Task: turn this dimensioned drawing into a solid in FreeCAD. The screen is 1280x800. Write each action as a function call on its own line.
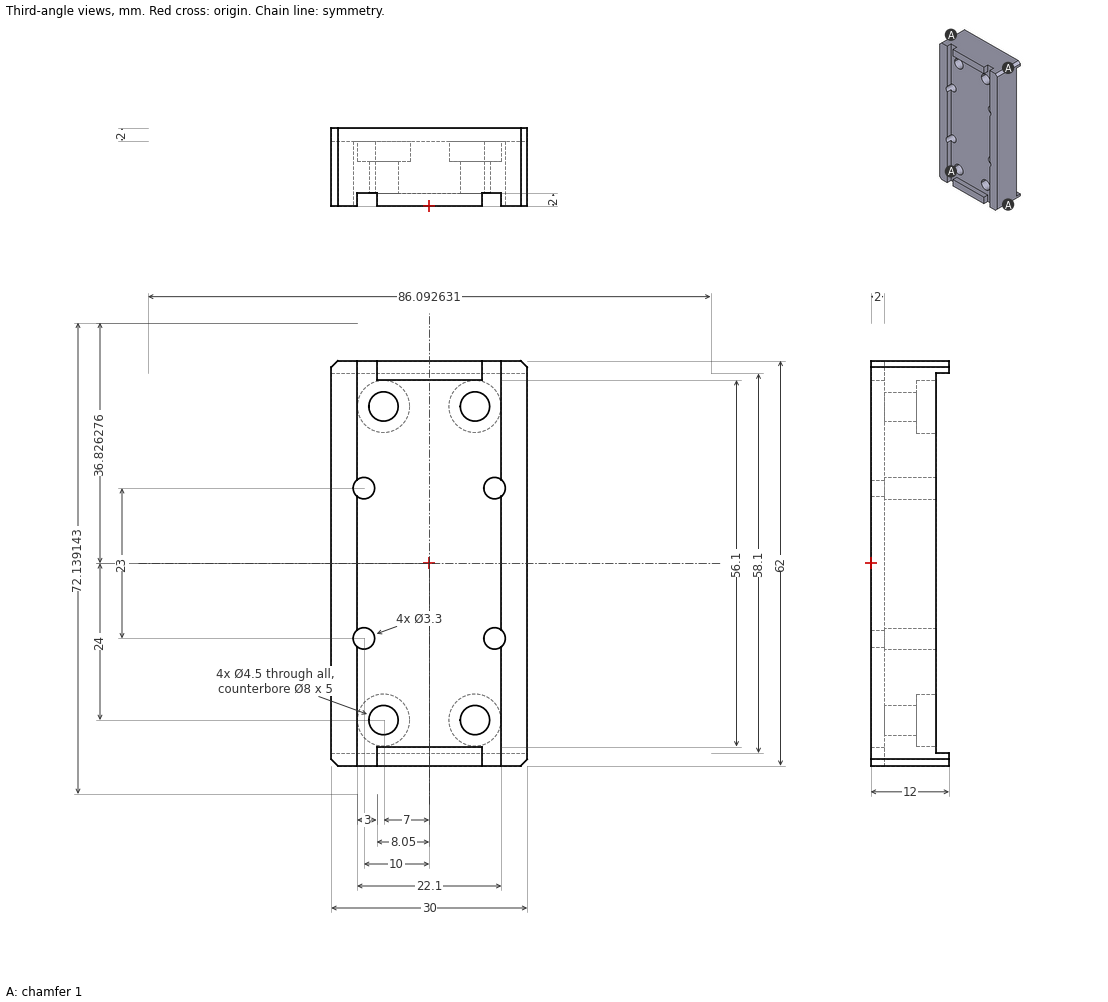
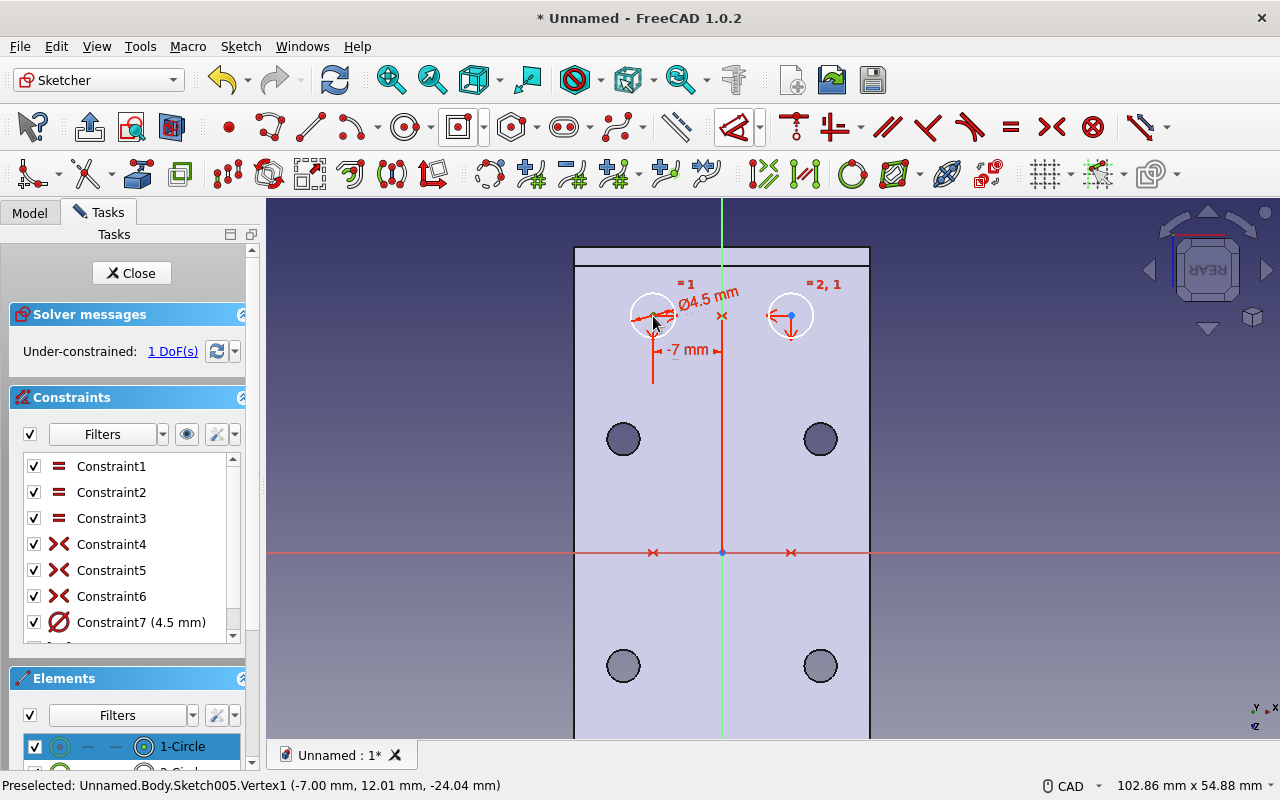
click(760, 128)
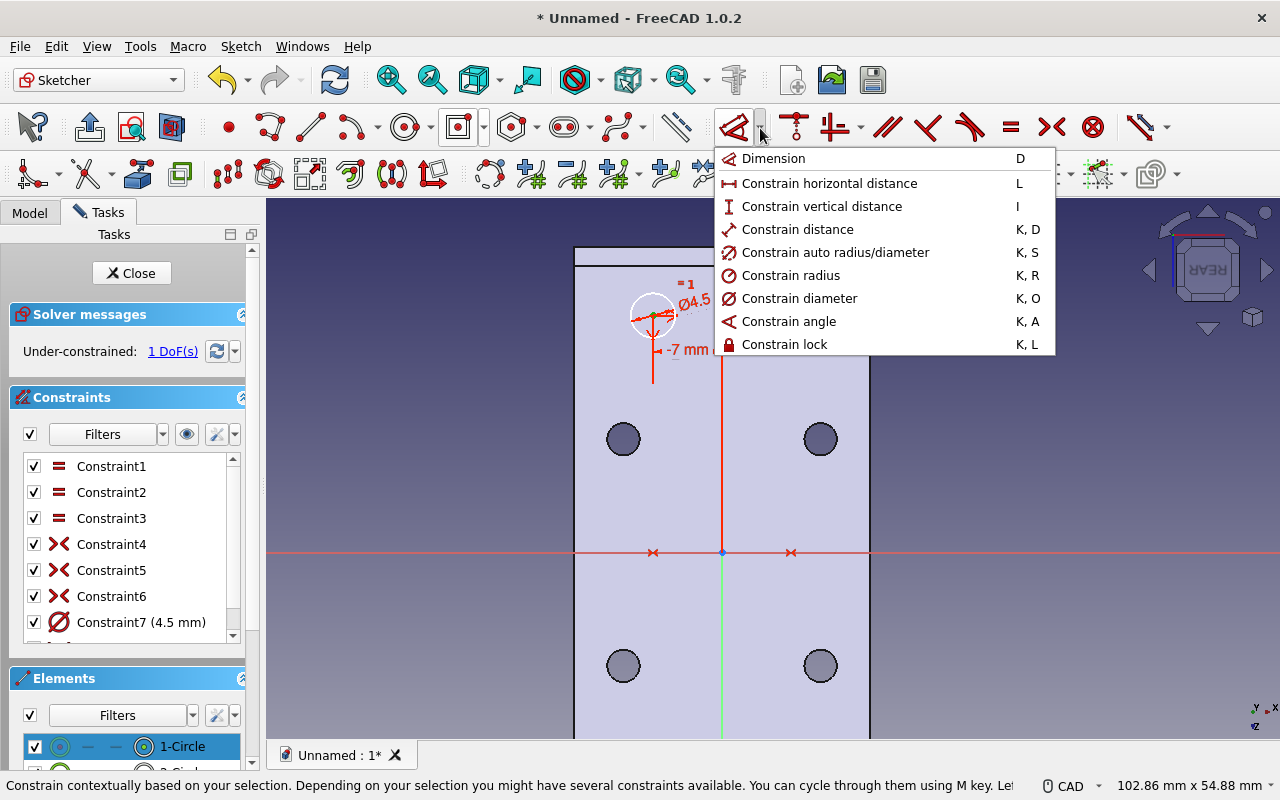
click(885, 206)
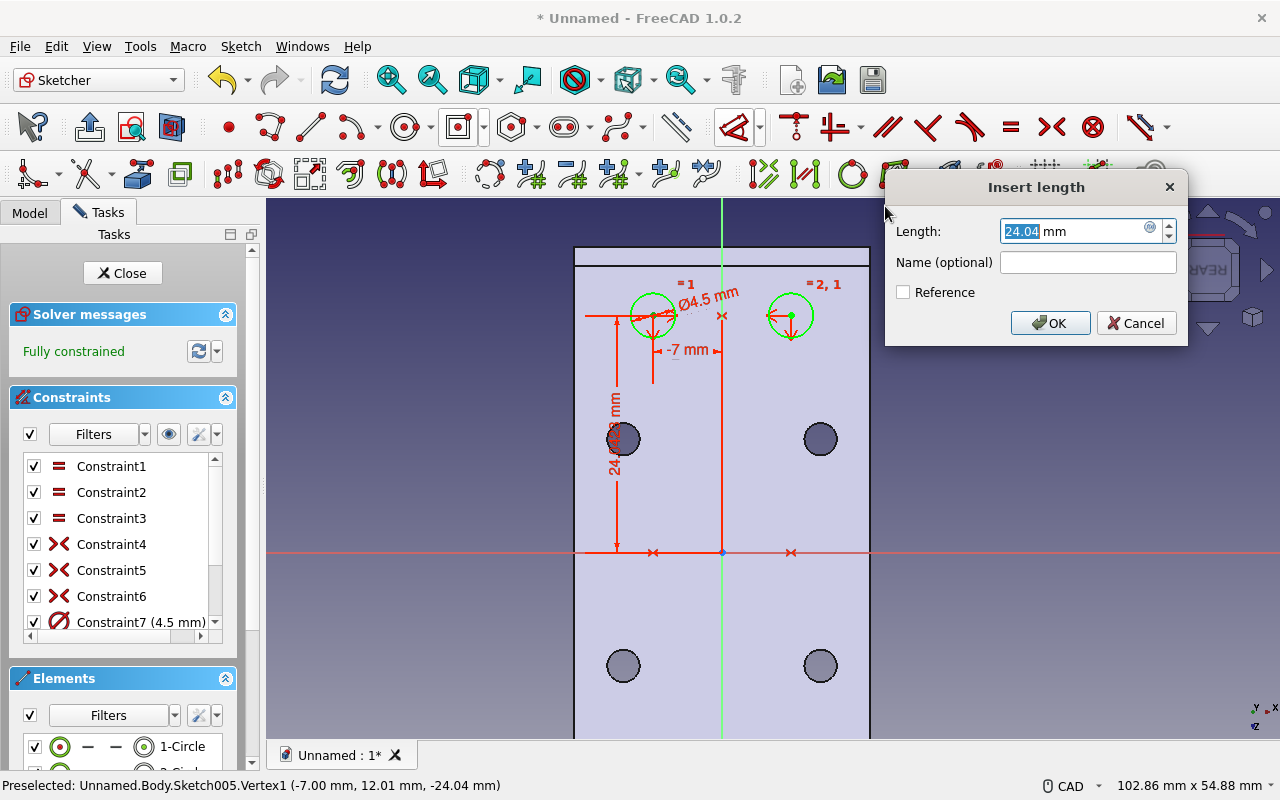
text(24)
key(Return)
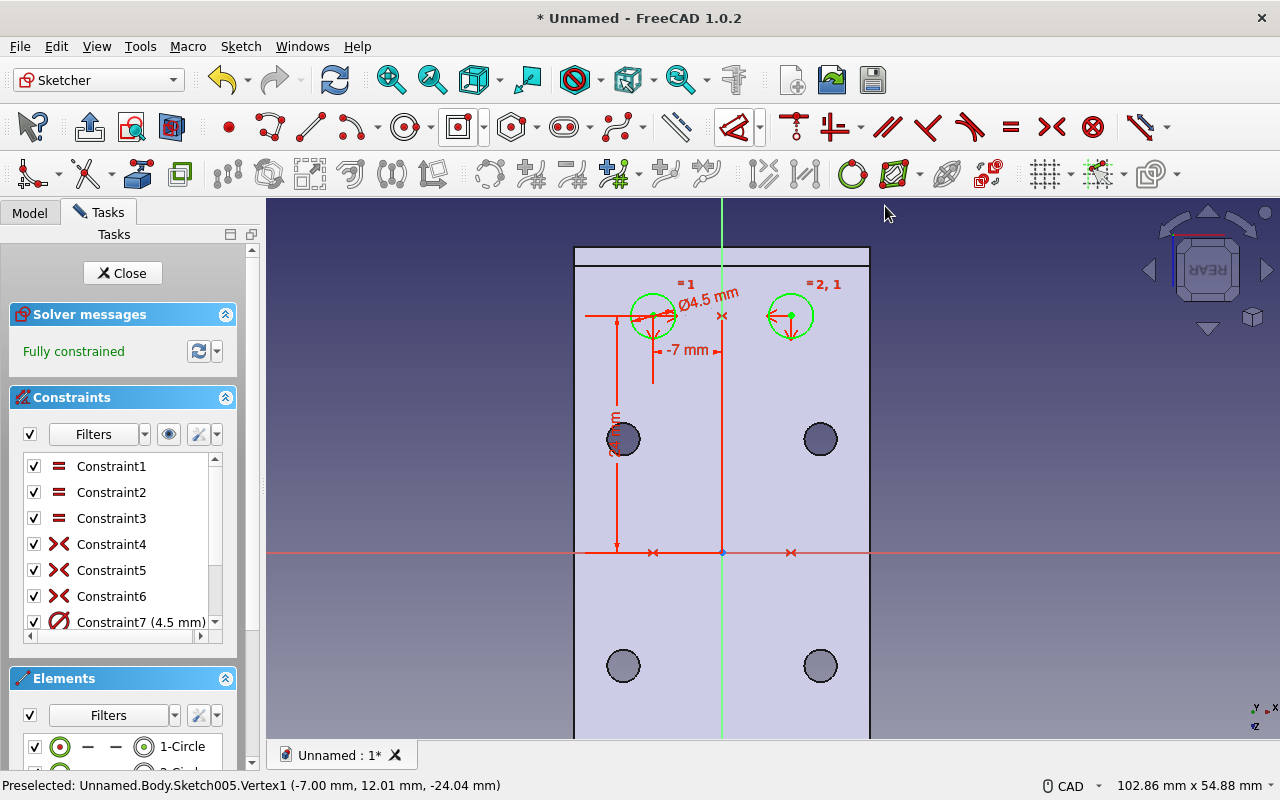
click(123, 273)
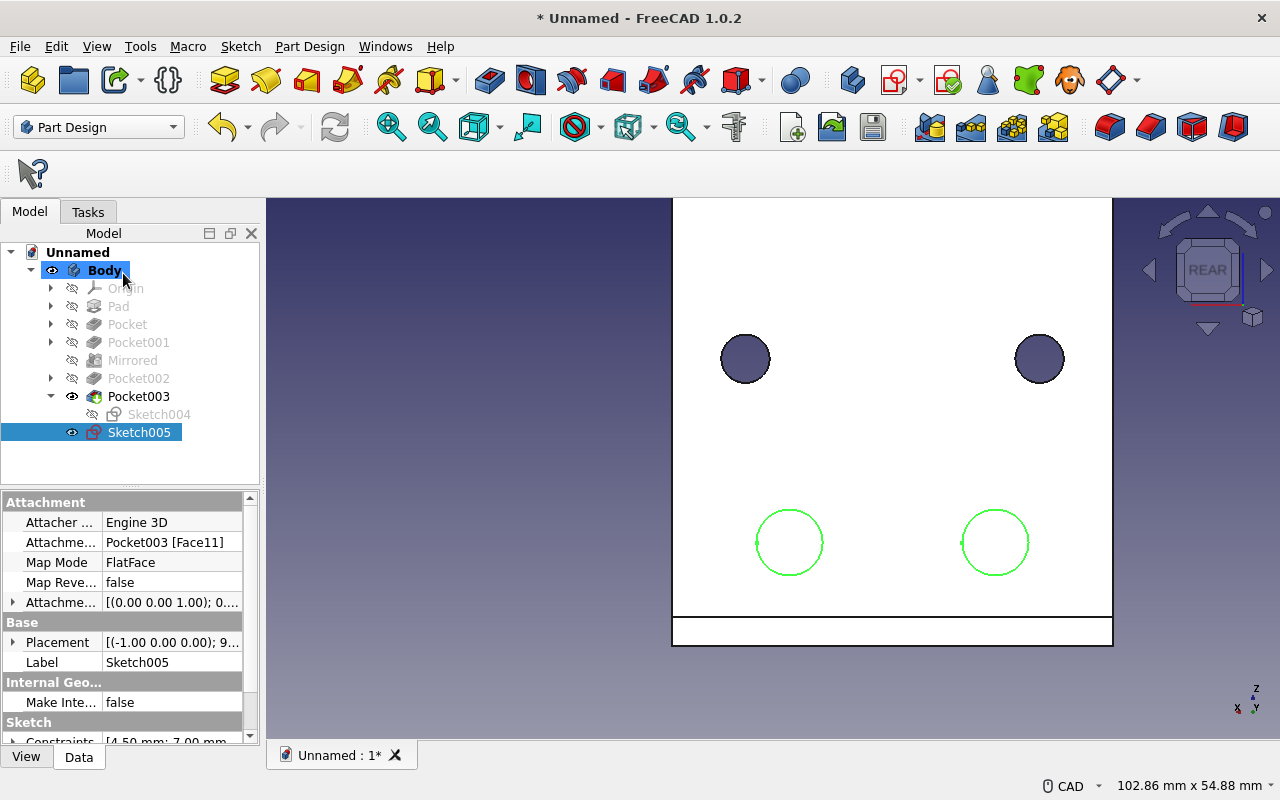
click(531, 80)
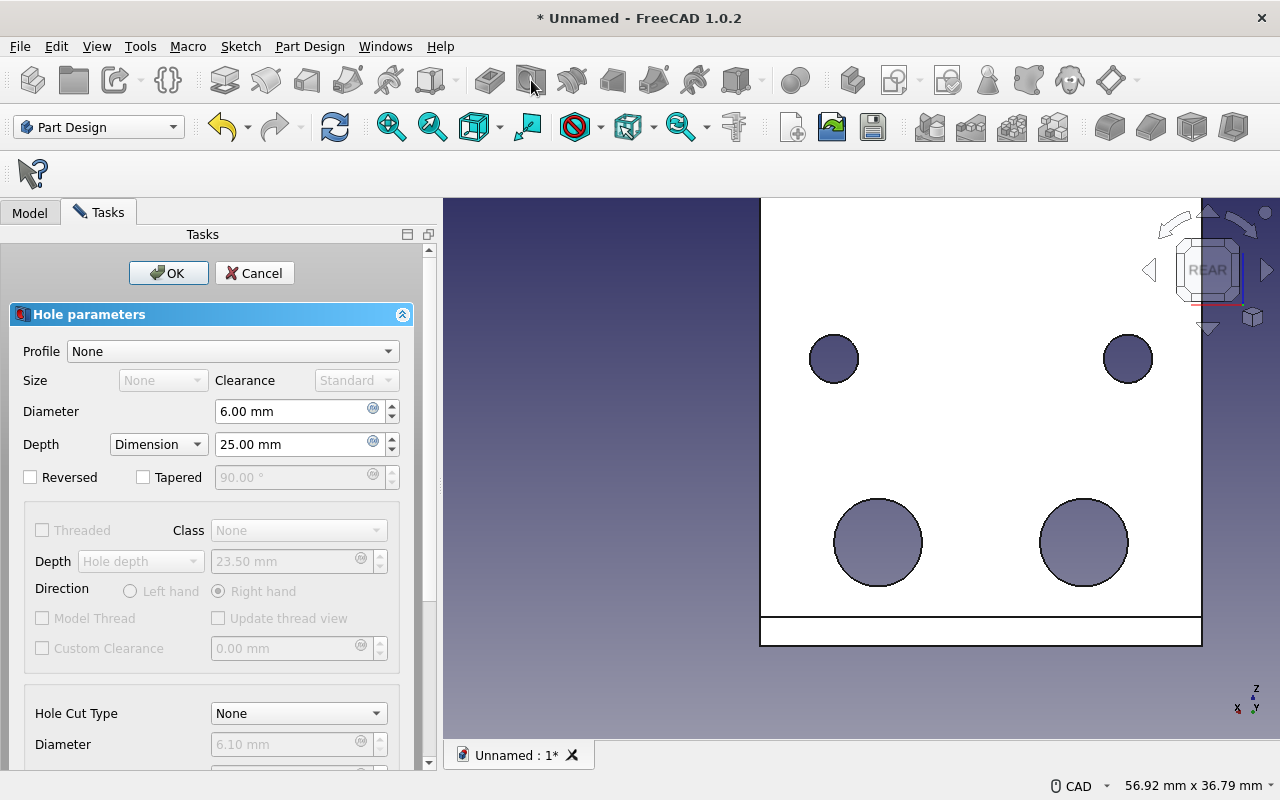
triple_click(300, 412)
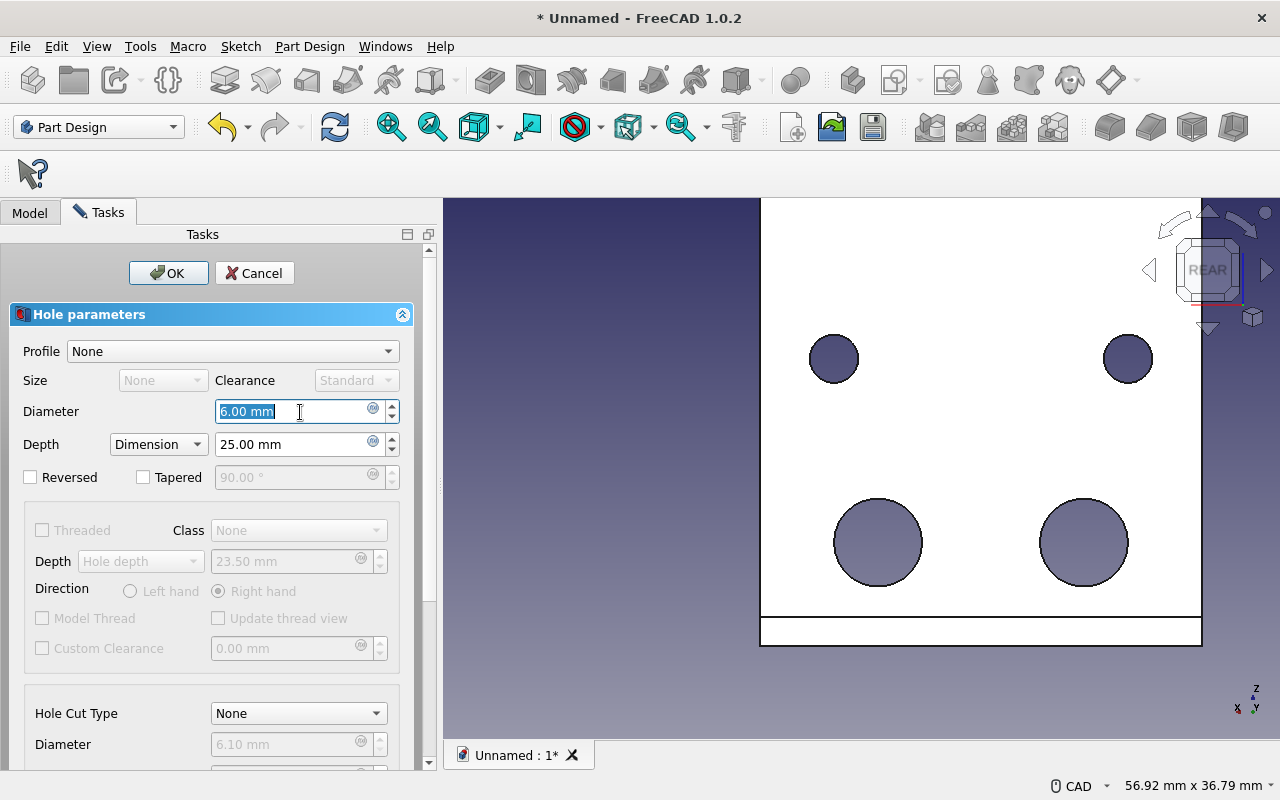
text(4.5)
key(Tab)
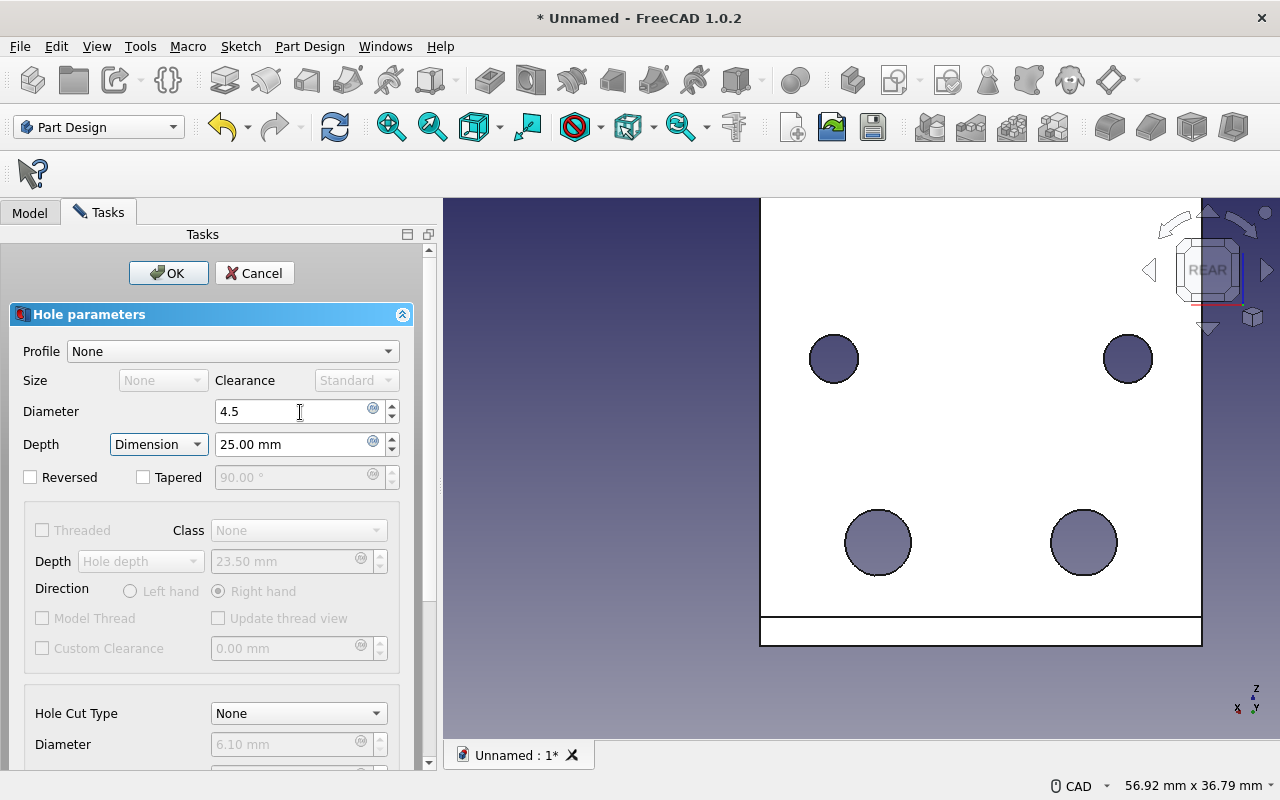
click(160, 444)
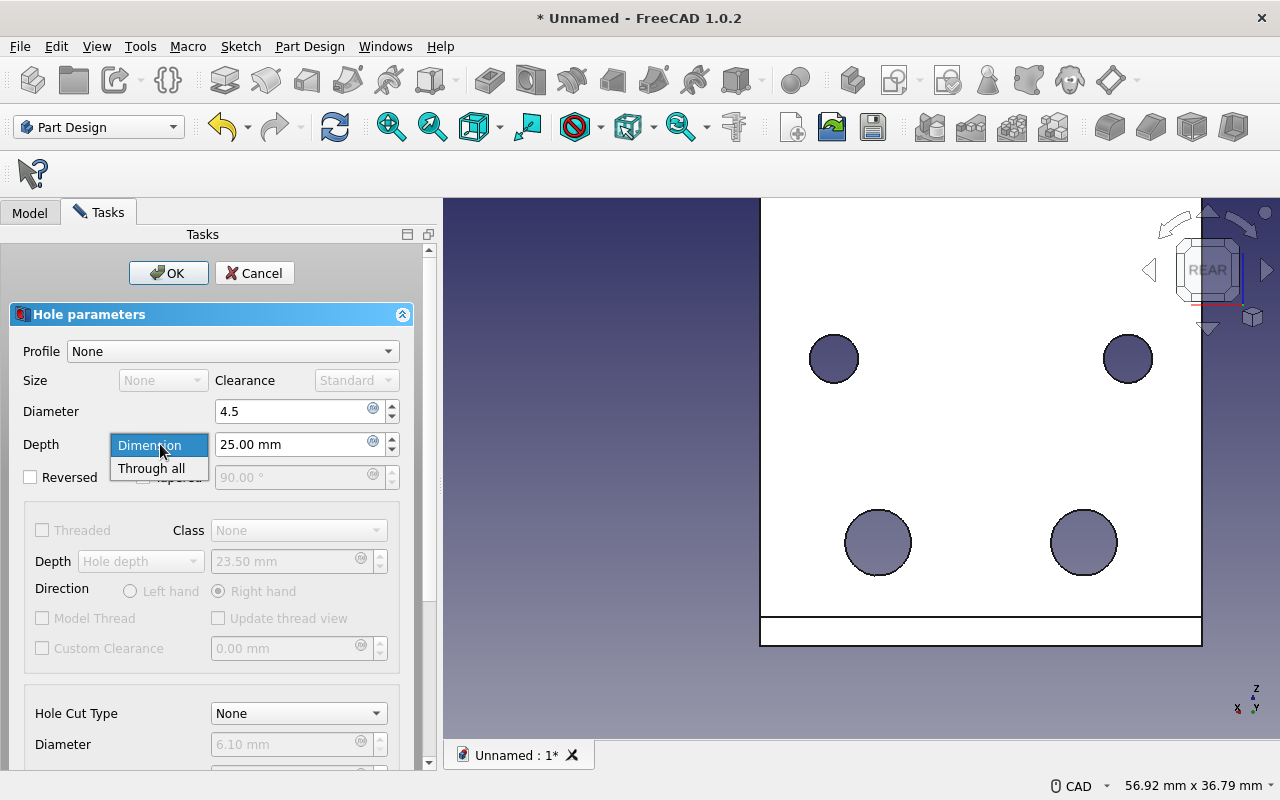
click(158, 468)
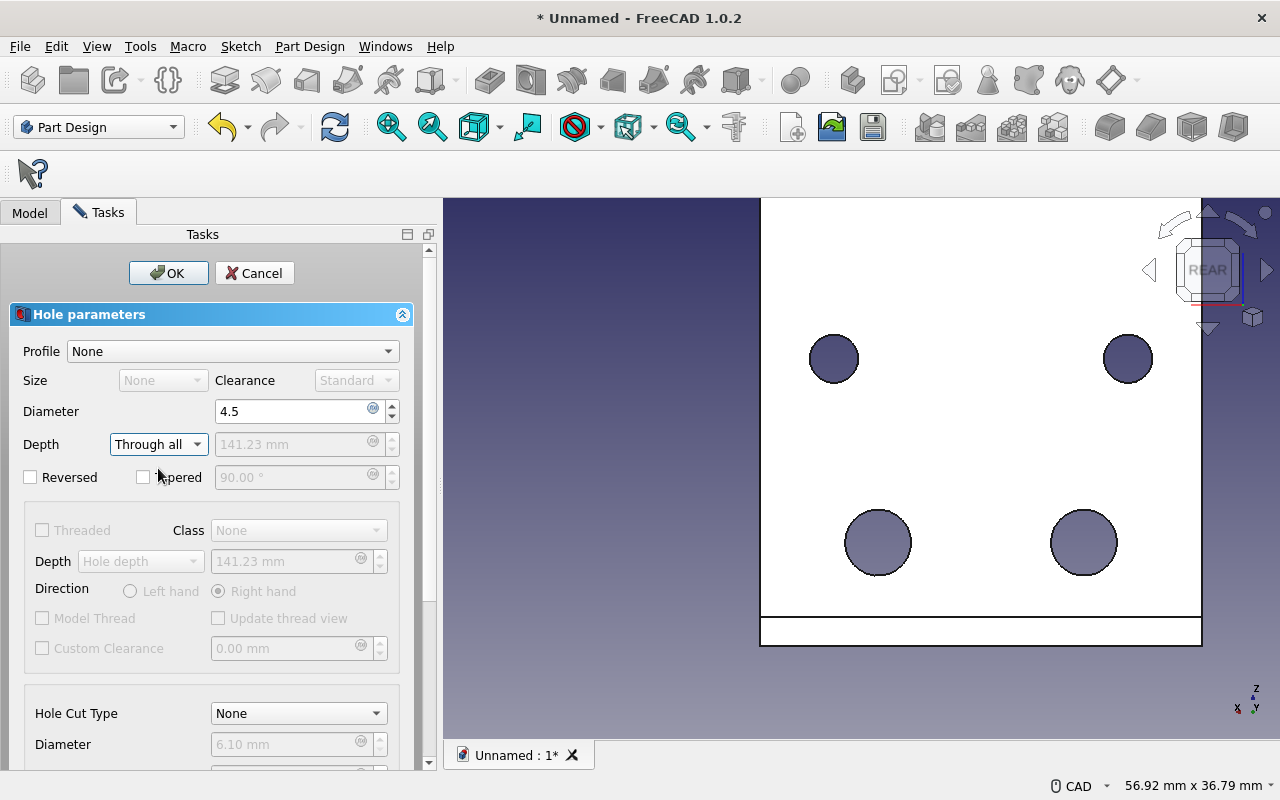
click(300, 714)